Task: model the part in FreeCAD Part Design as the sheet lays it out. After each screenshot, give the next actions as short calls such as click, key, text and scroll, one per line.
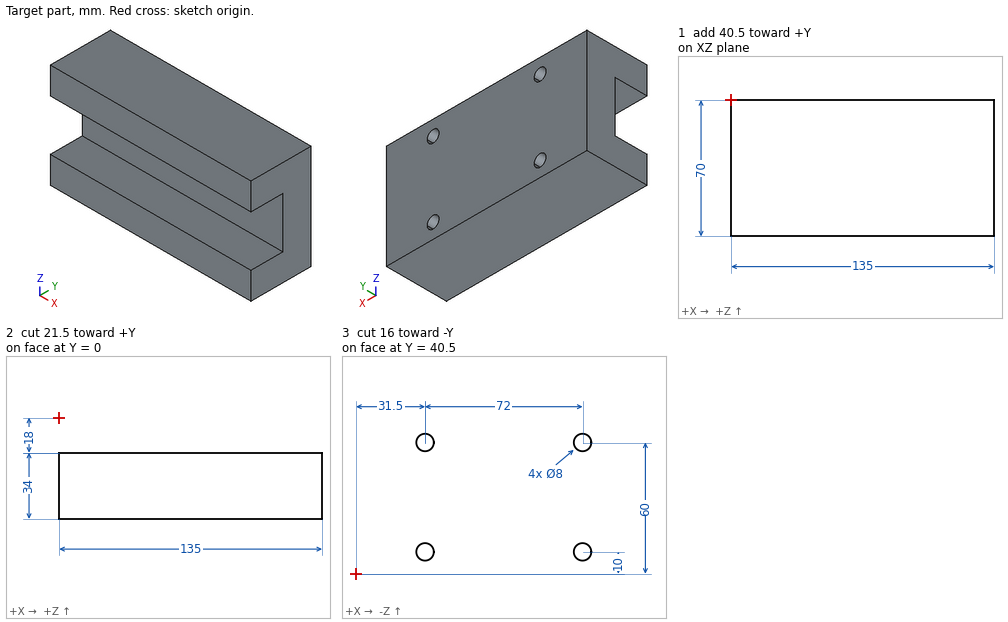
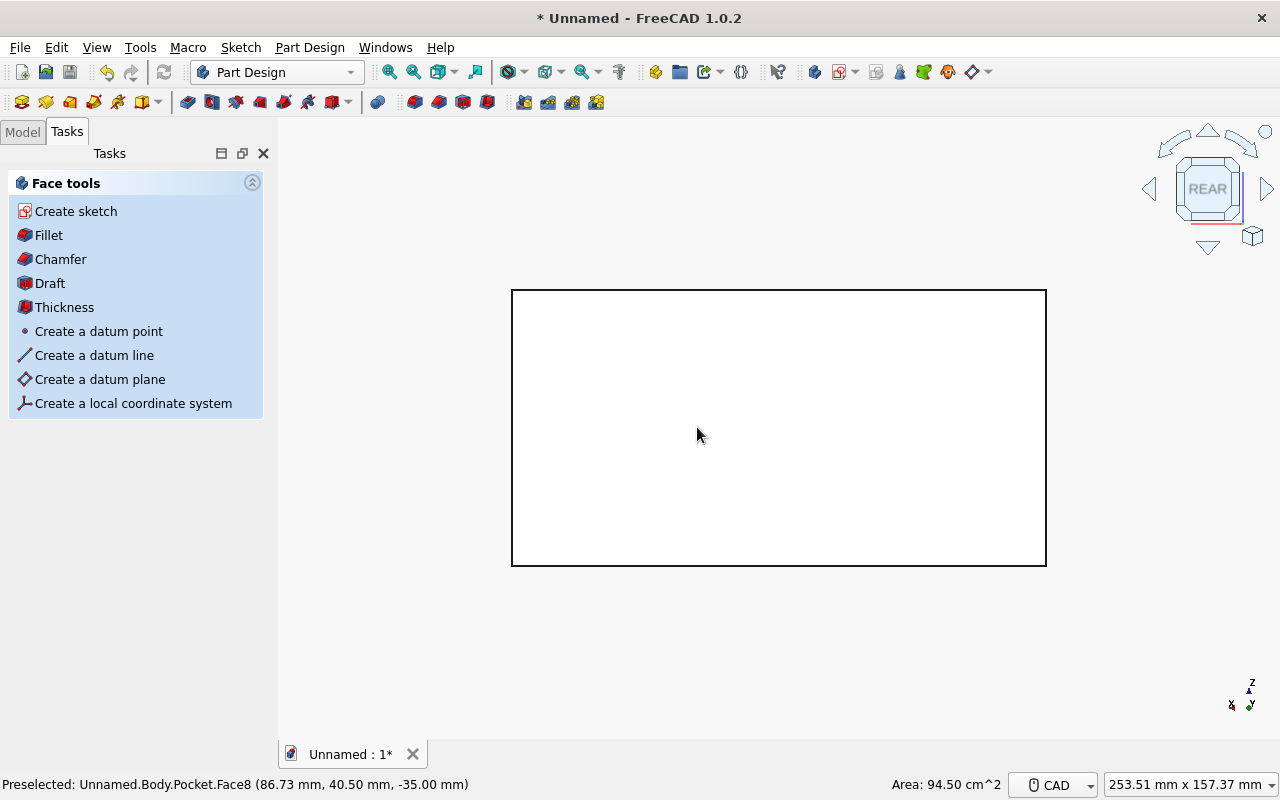
click(840, 72)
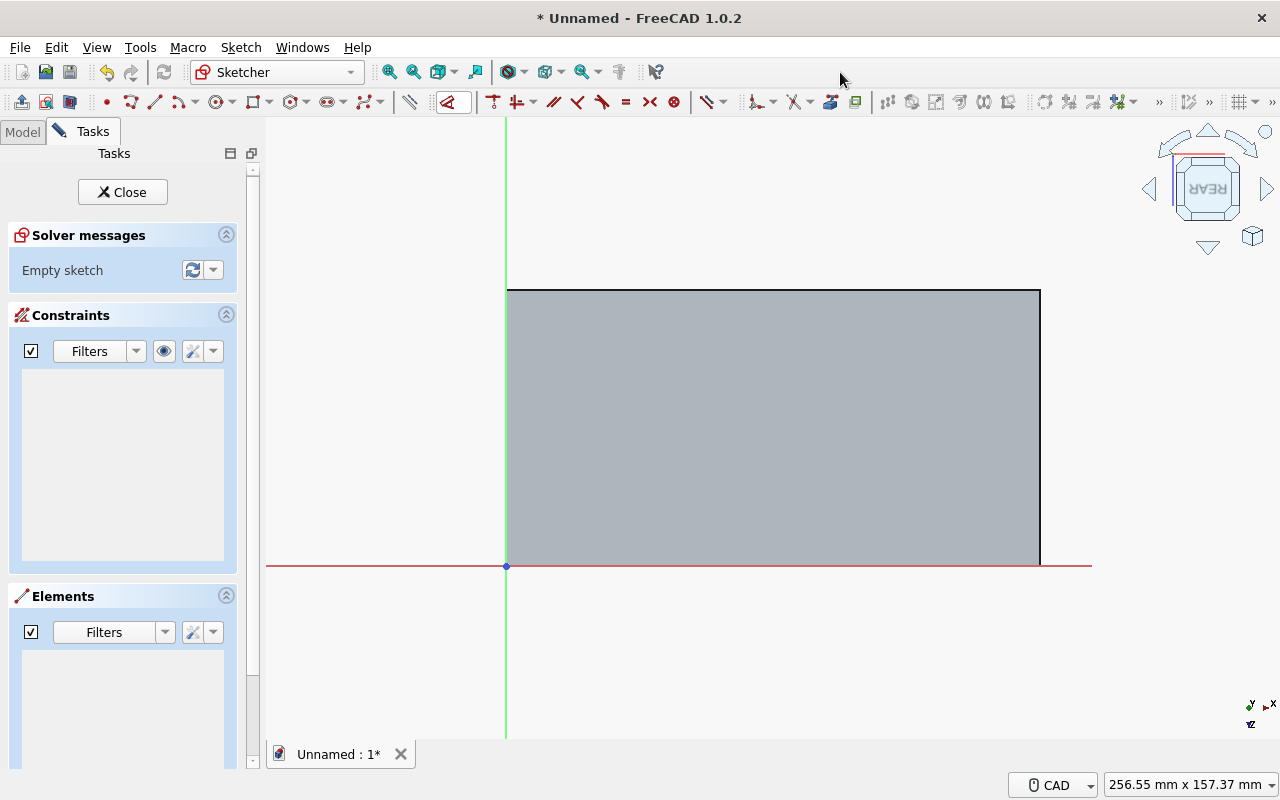
scroll(747, 464, up, 2)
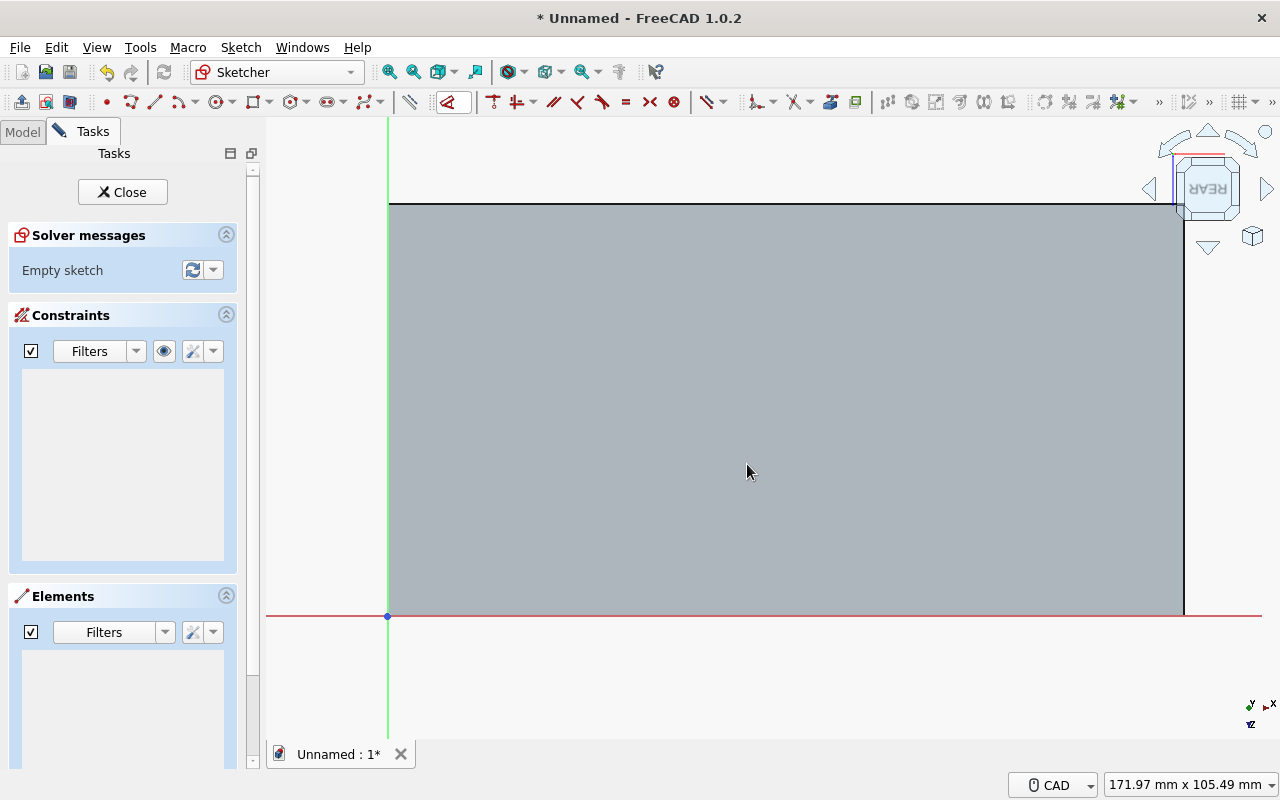
click(216, 102)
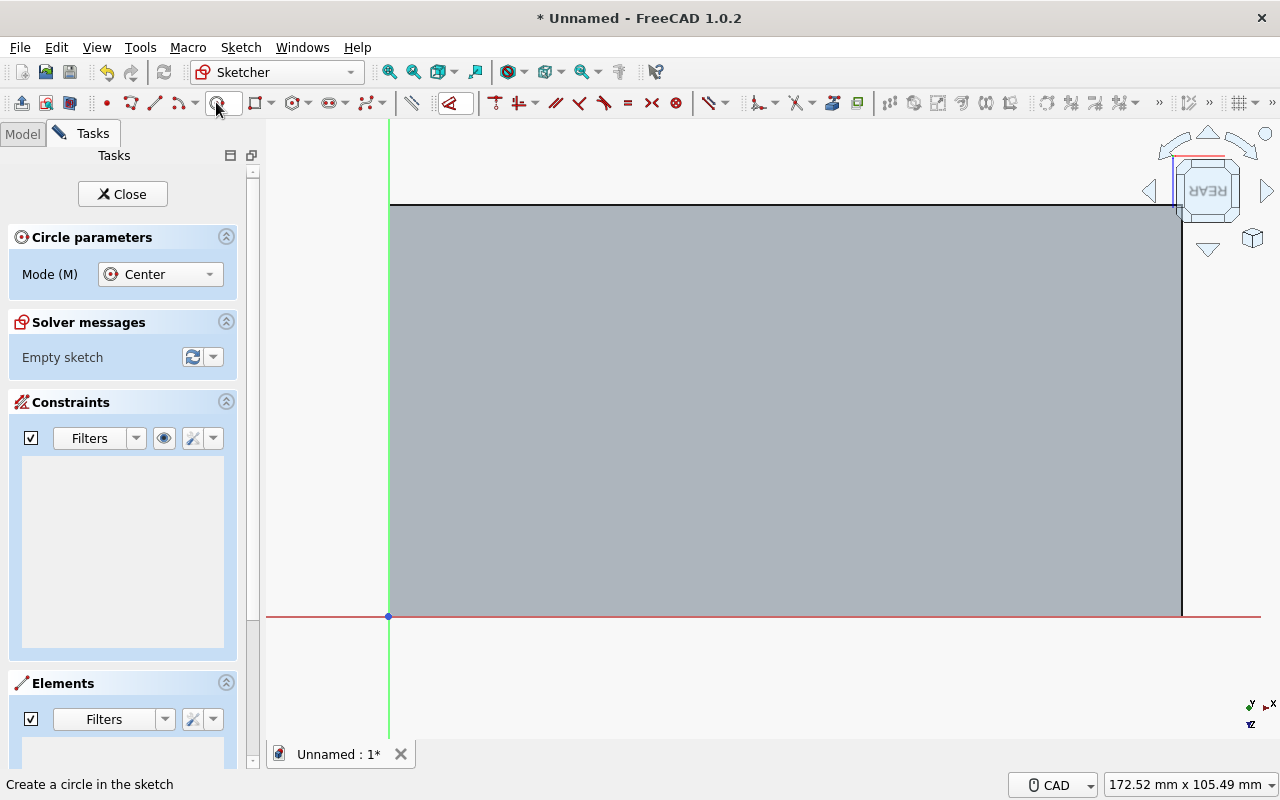
click(997, 264)
click(1014, 248)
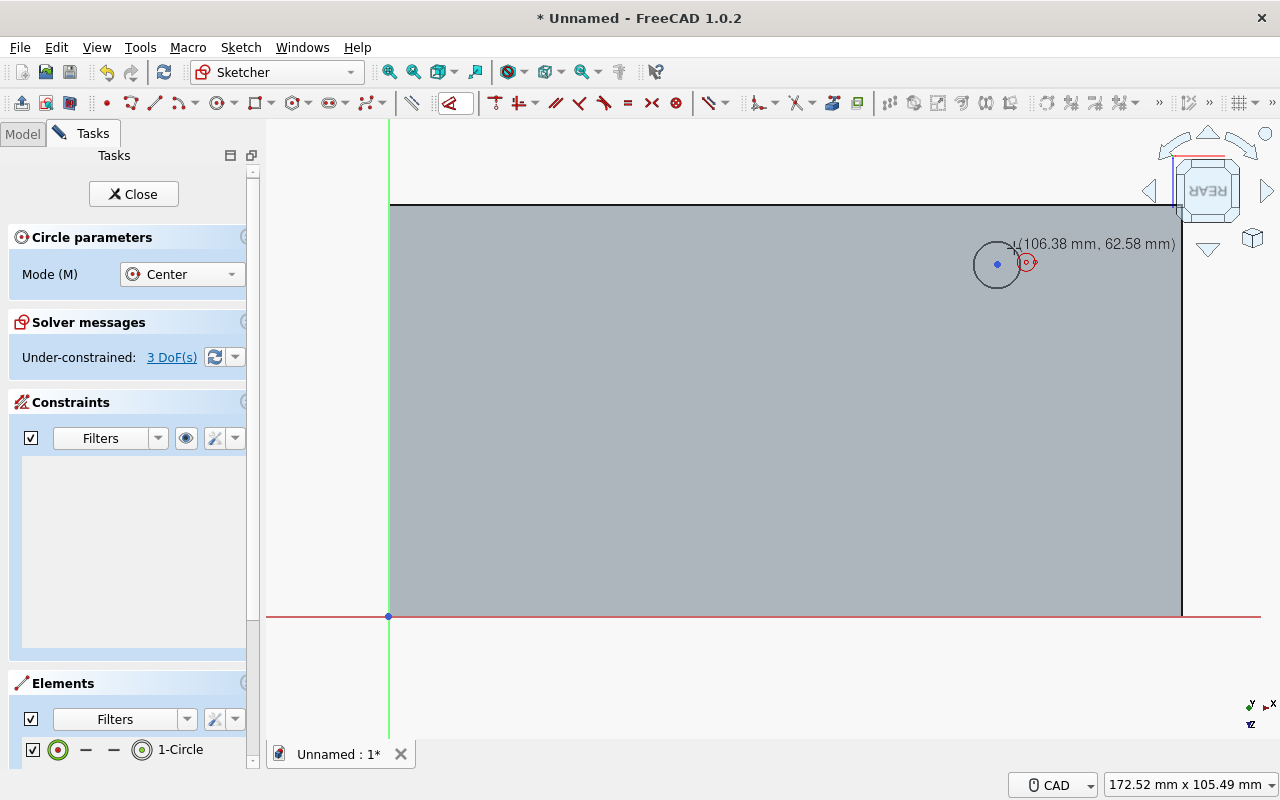
click(997, 558)
click(1014, 541)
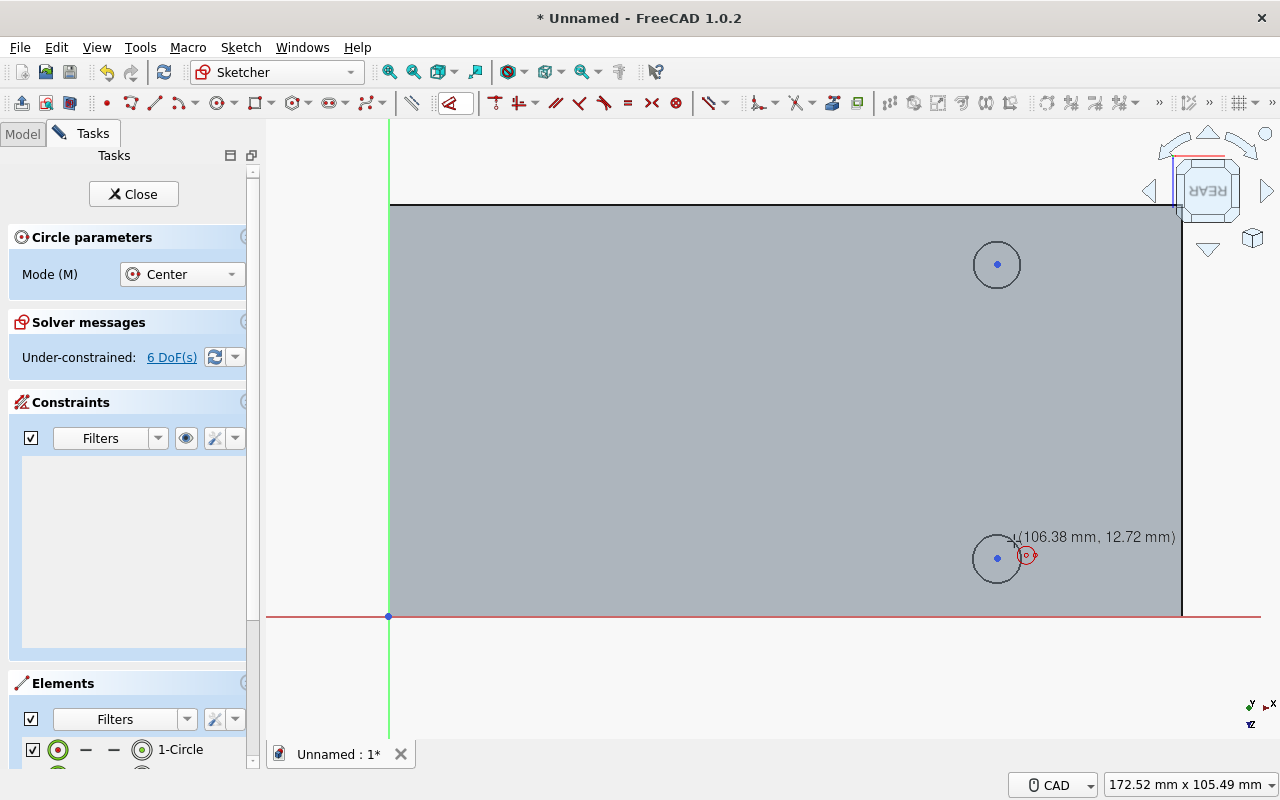
click(574, 264)
click(591, 248)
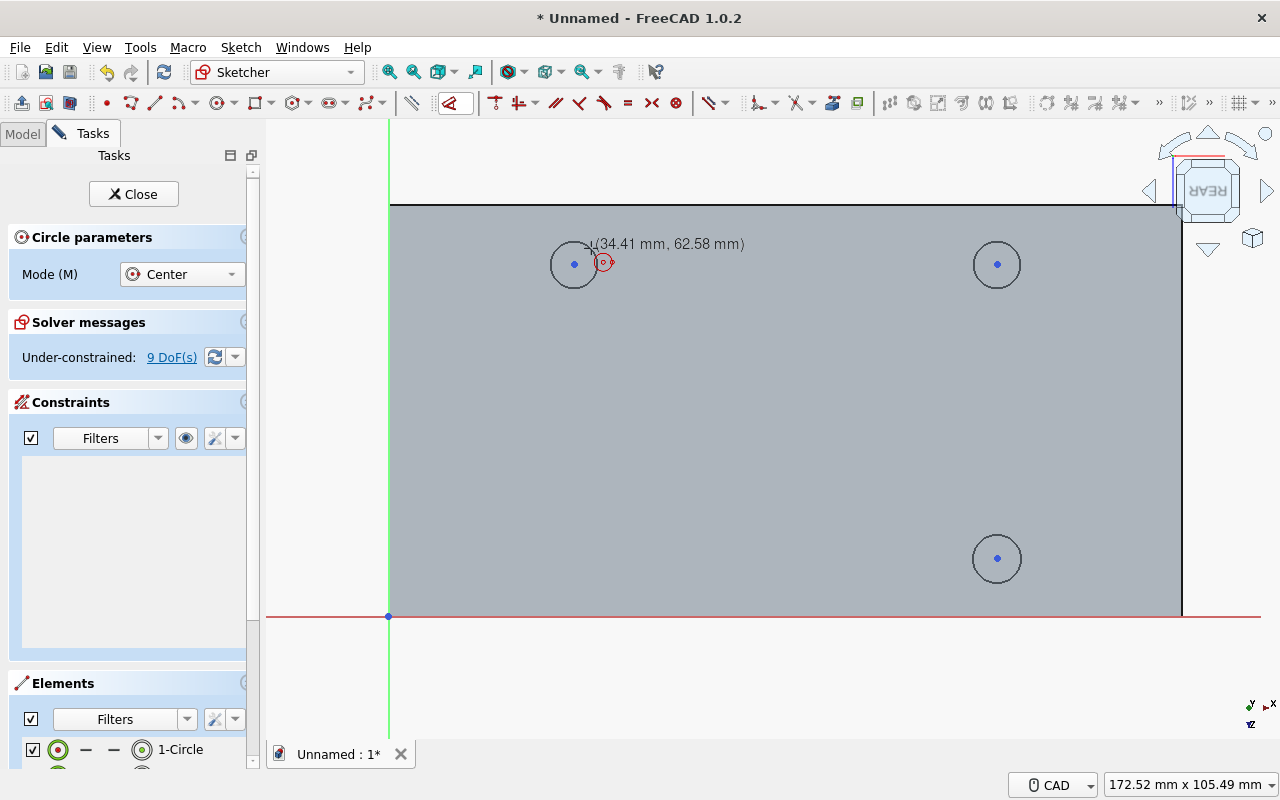
click(574, 558)
click(591, 541)
key(Escape)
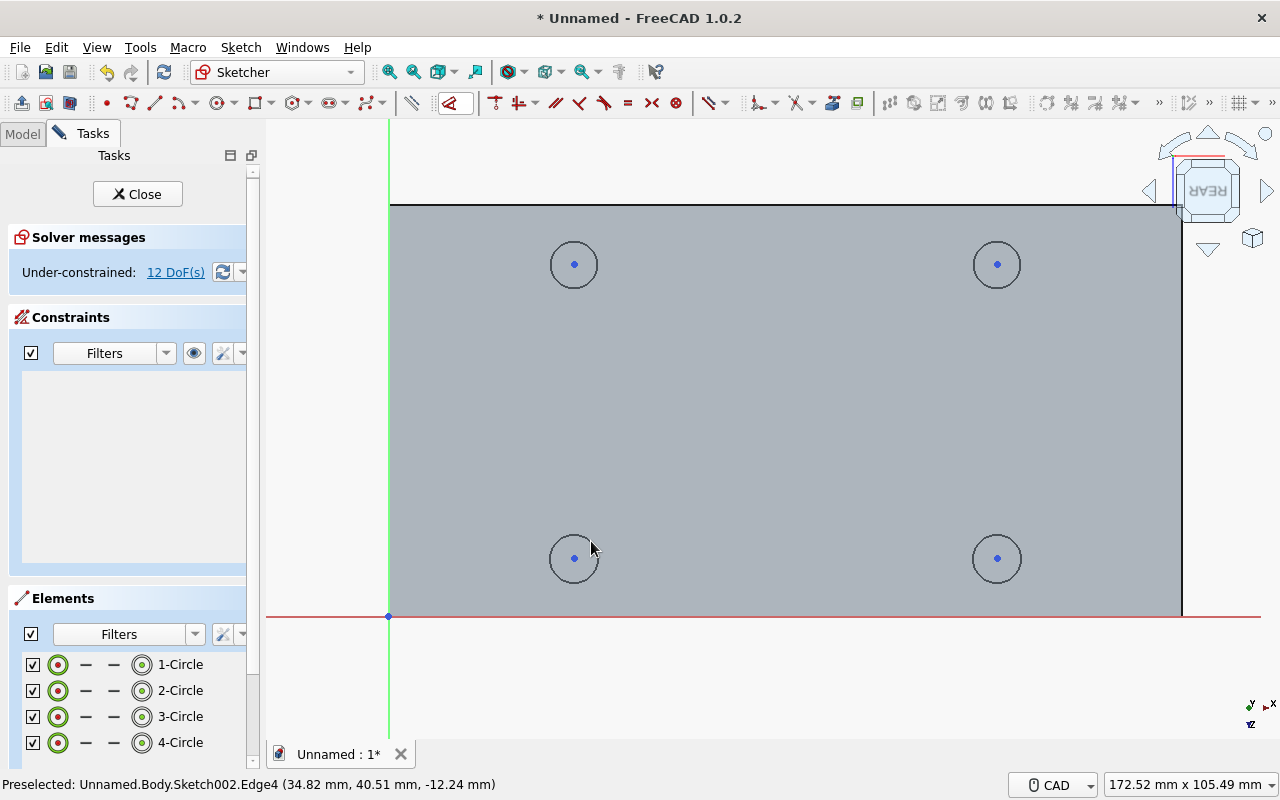
click(1013, 248)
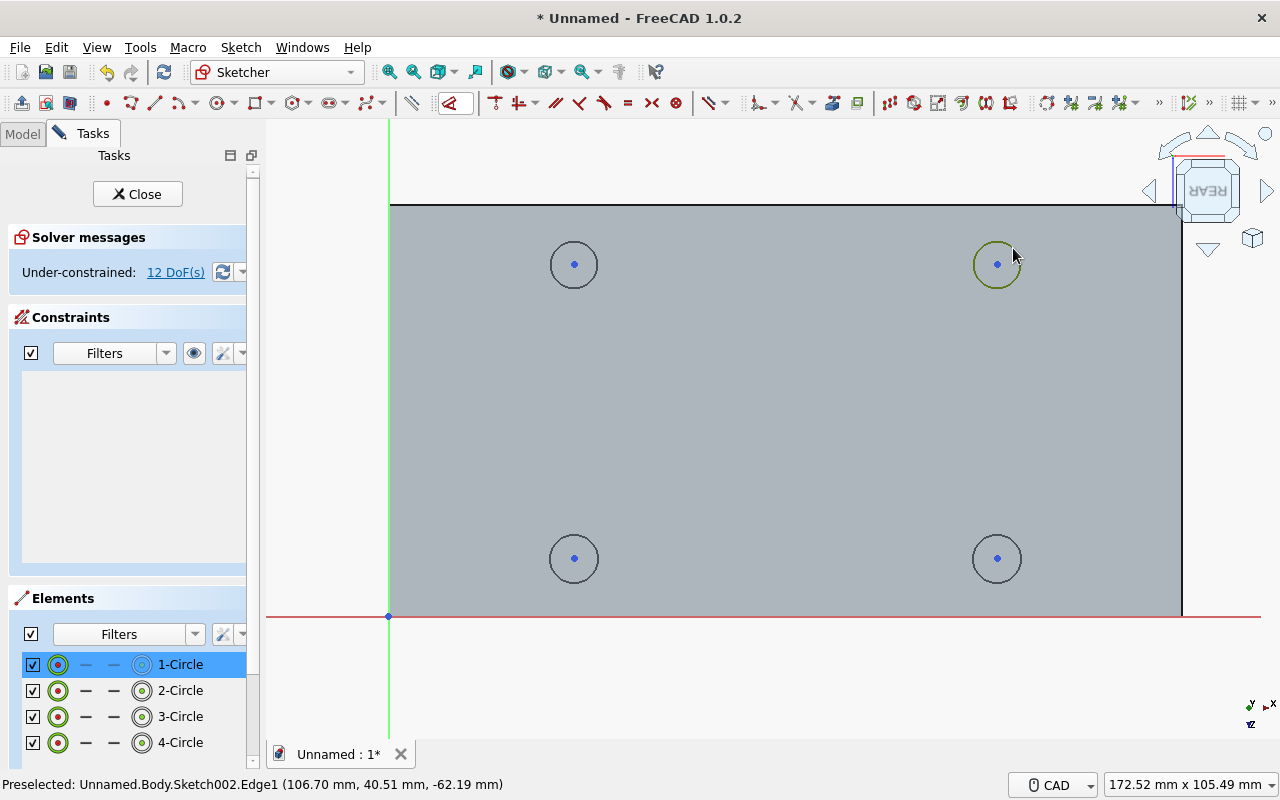
click(1014, 542)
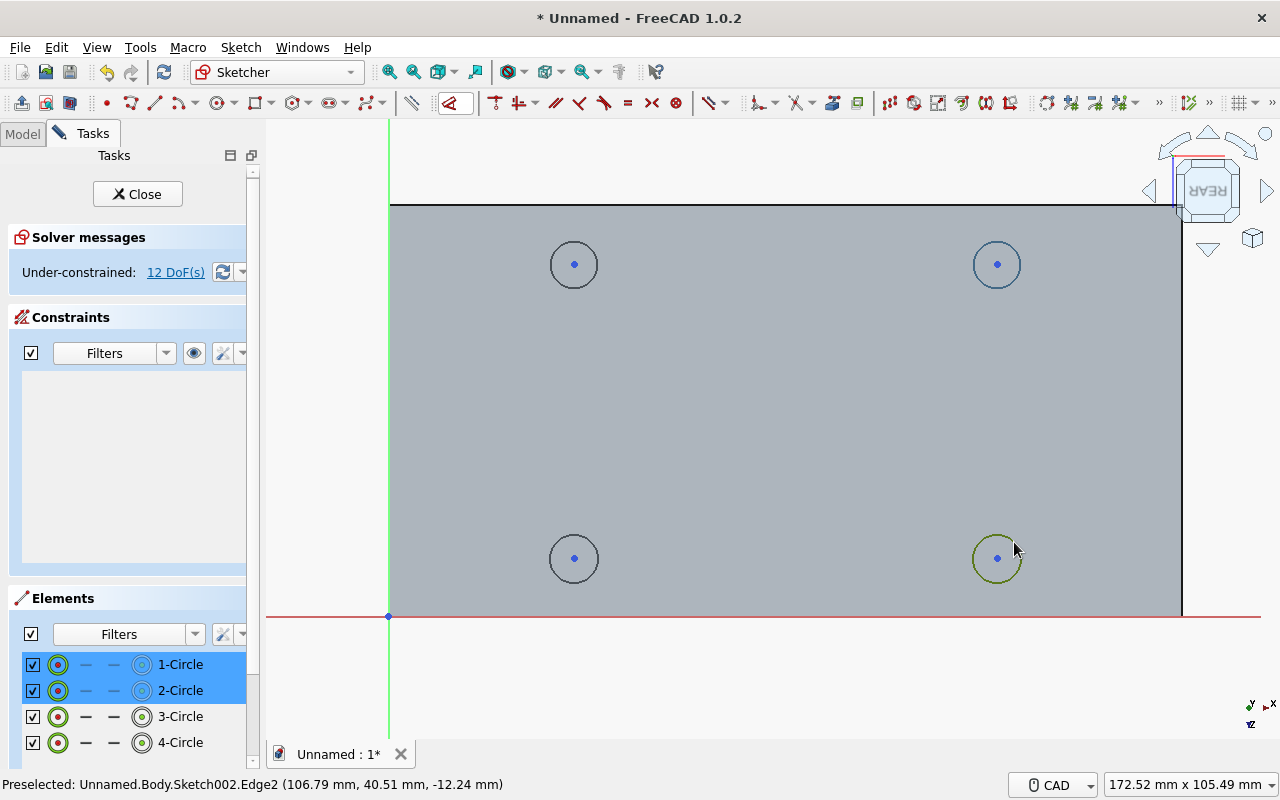
click(590, 248)